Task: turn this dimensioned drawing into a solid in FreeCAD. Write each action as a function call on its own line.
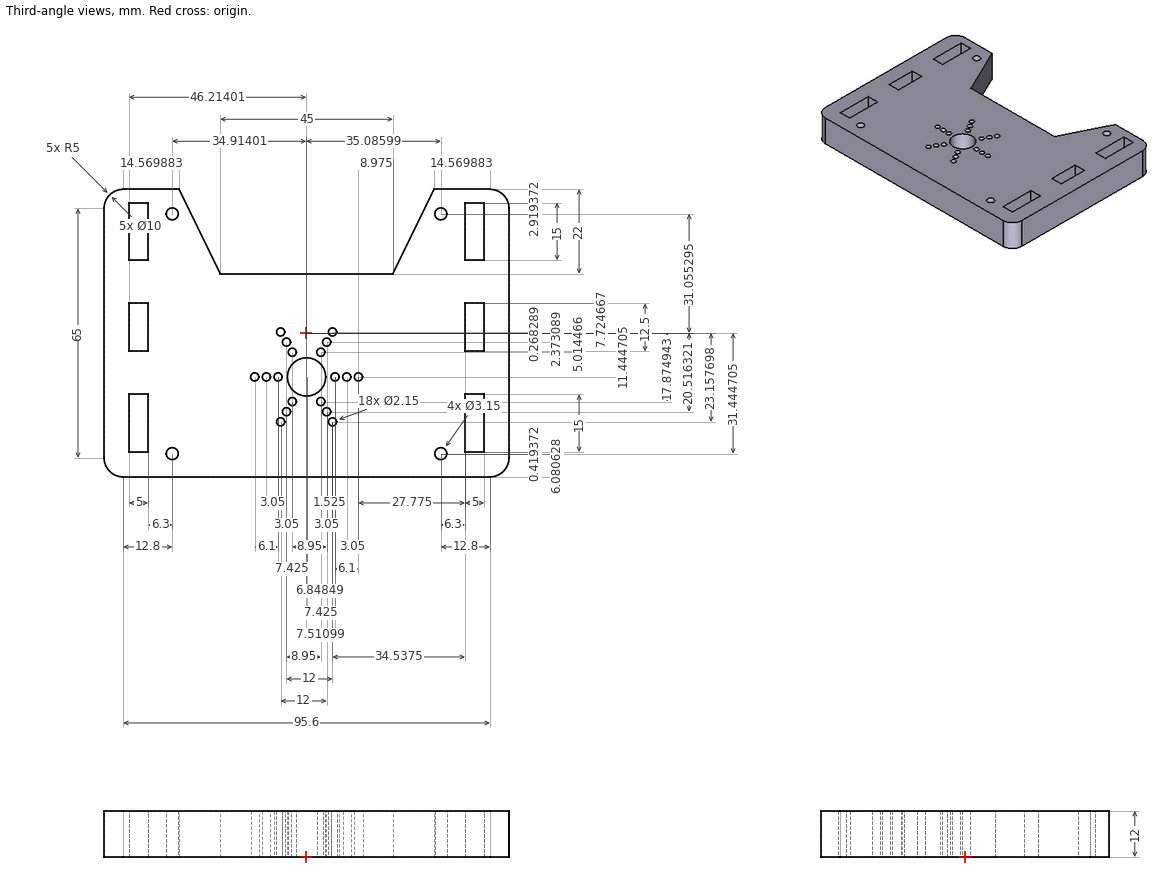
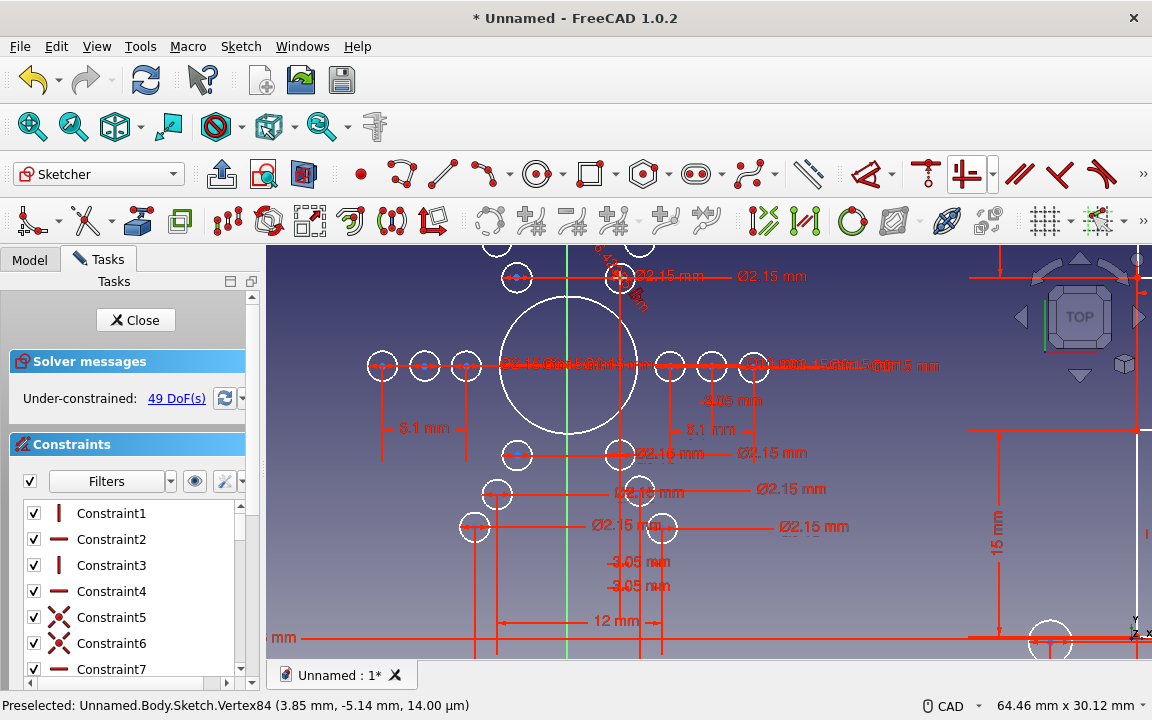
scroll(664, 532, down, 7)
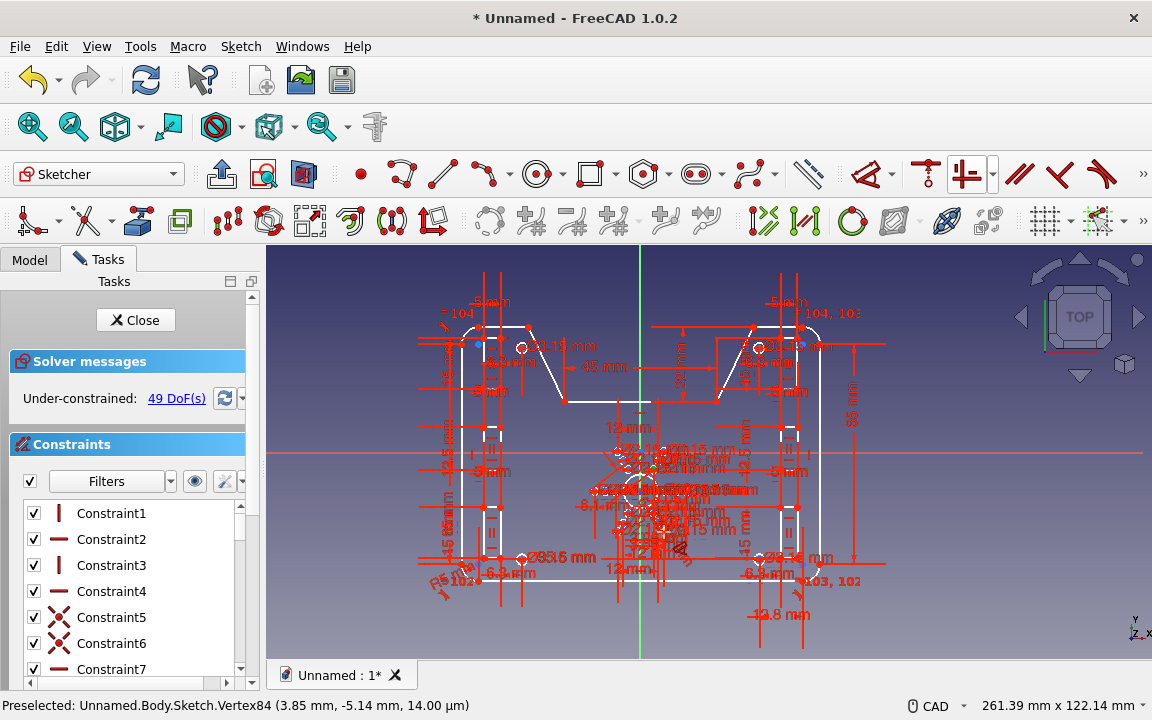
scroll(664, 452, up, 7)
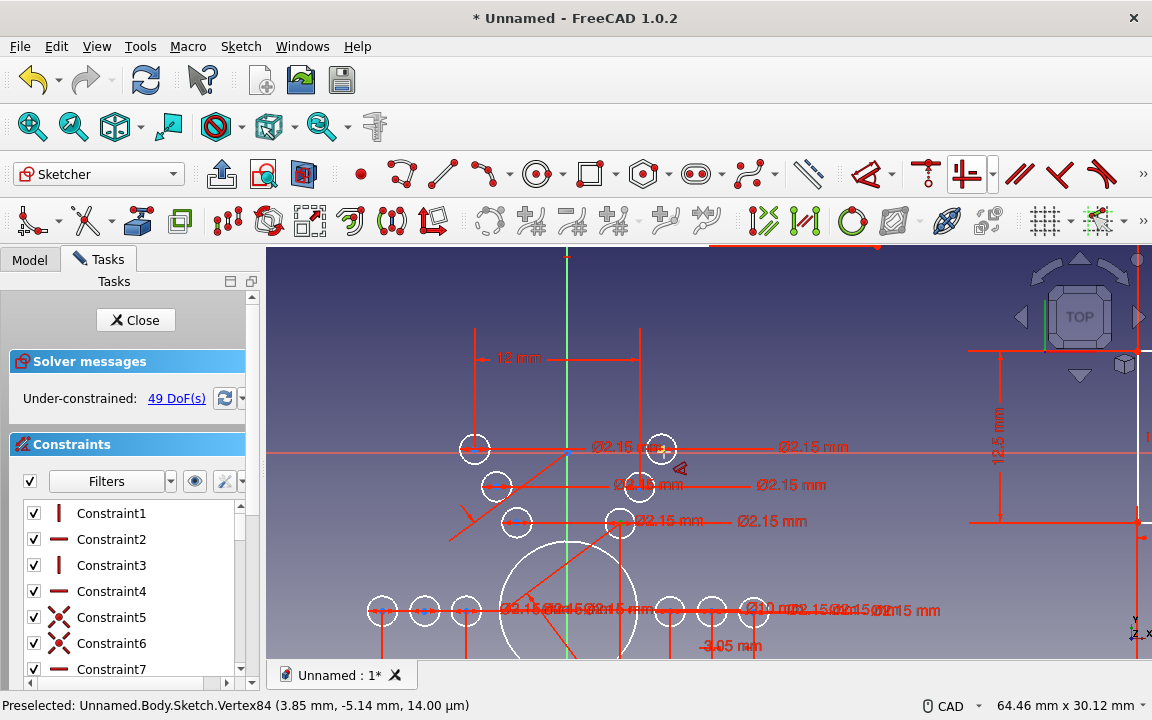
click(661, 449)
click(641, 557)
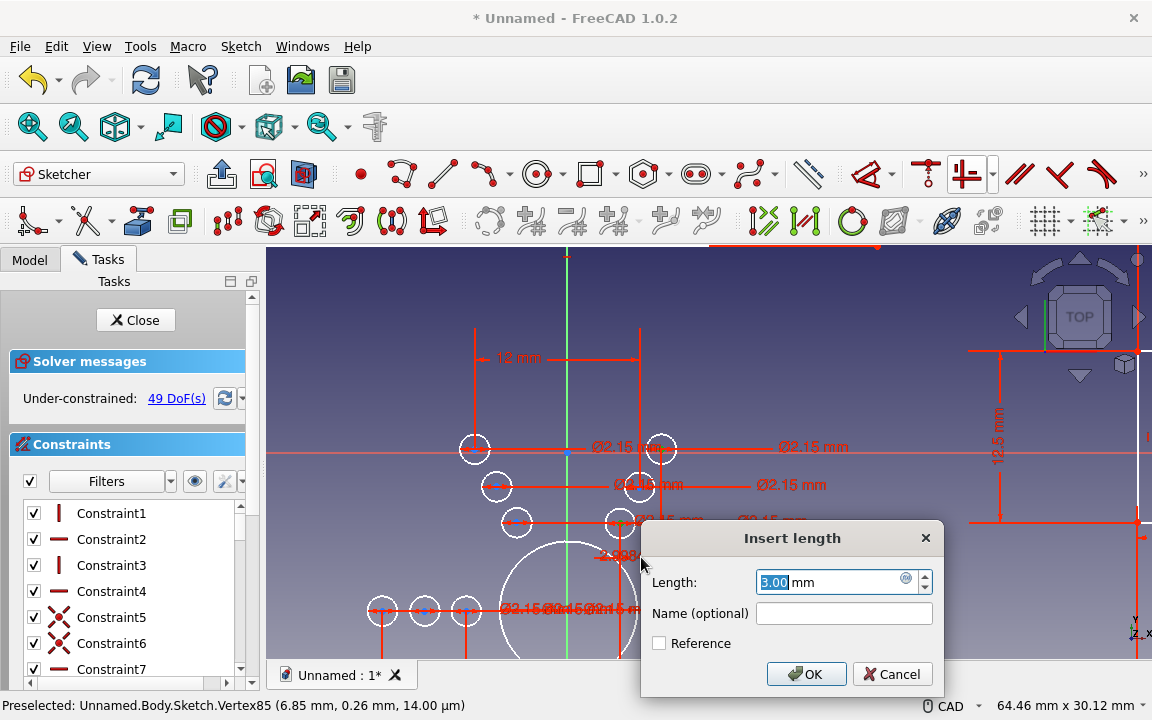
text(3.05)
key(Return)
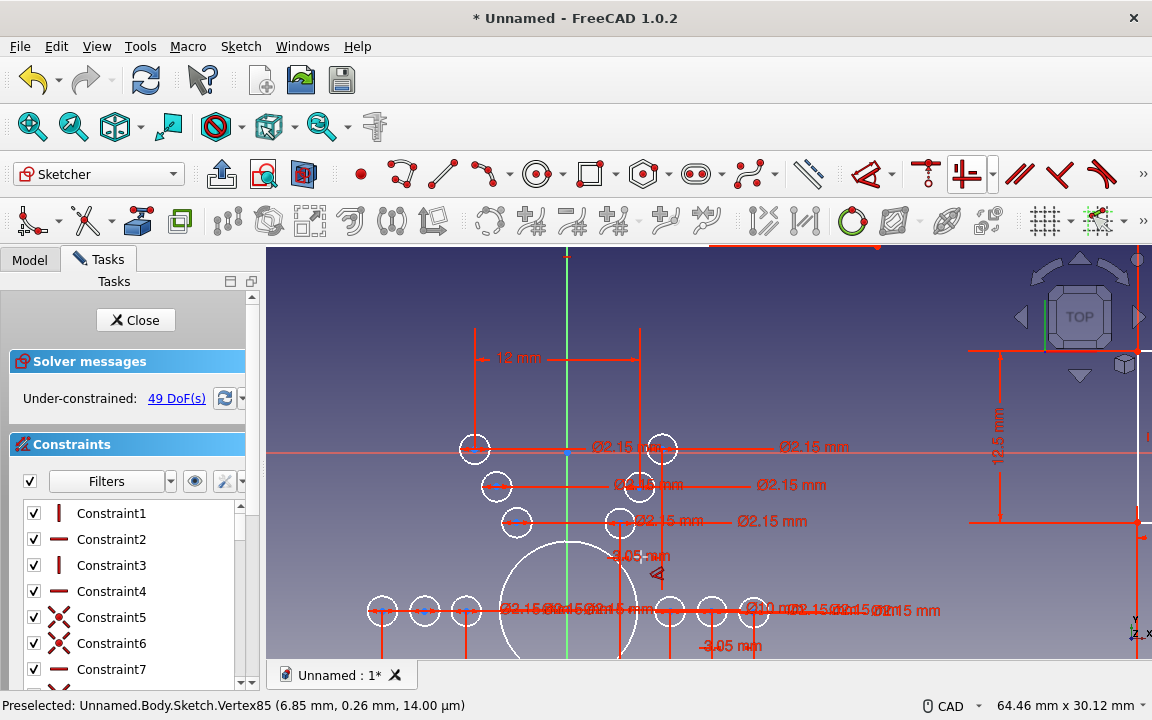
scroll(664, 452, down, 7)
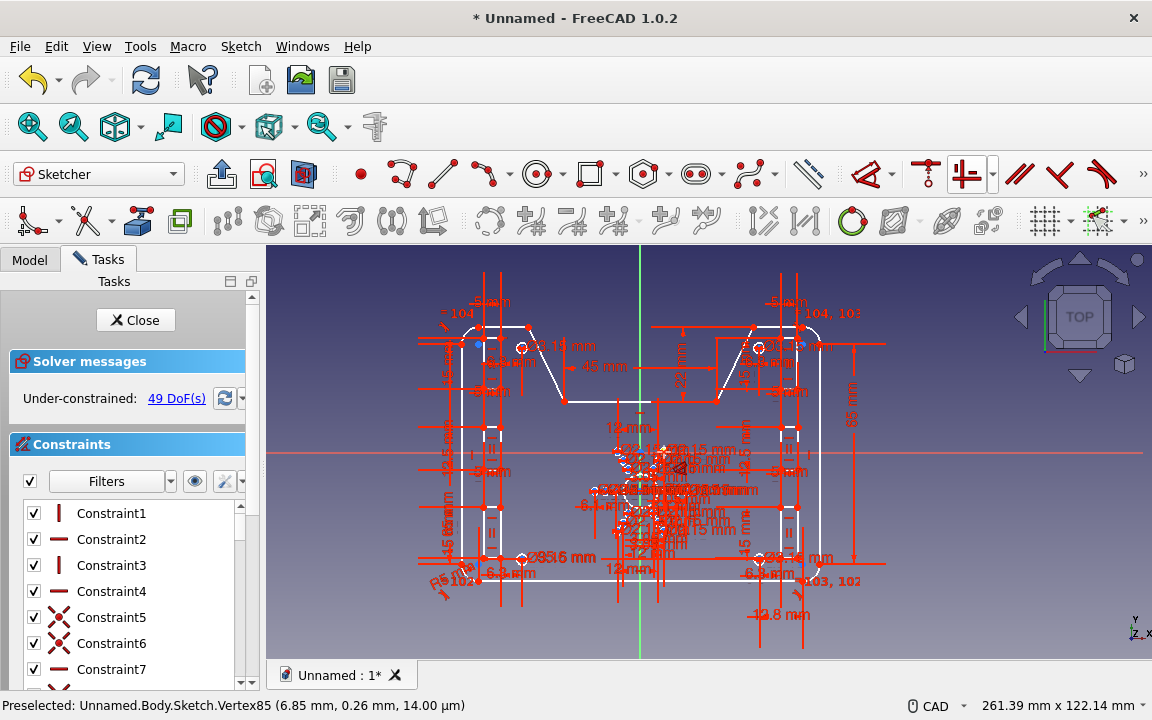
scroll(618, 531, up, 7)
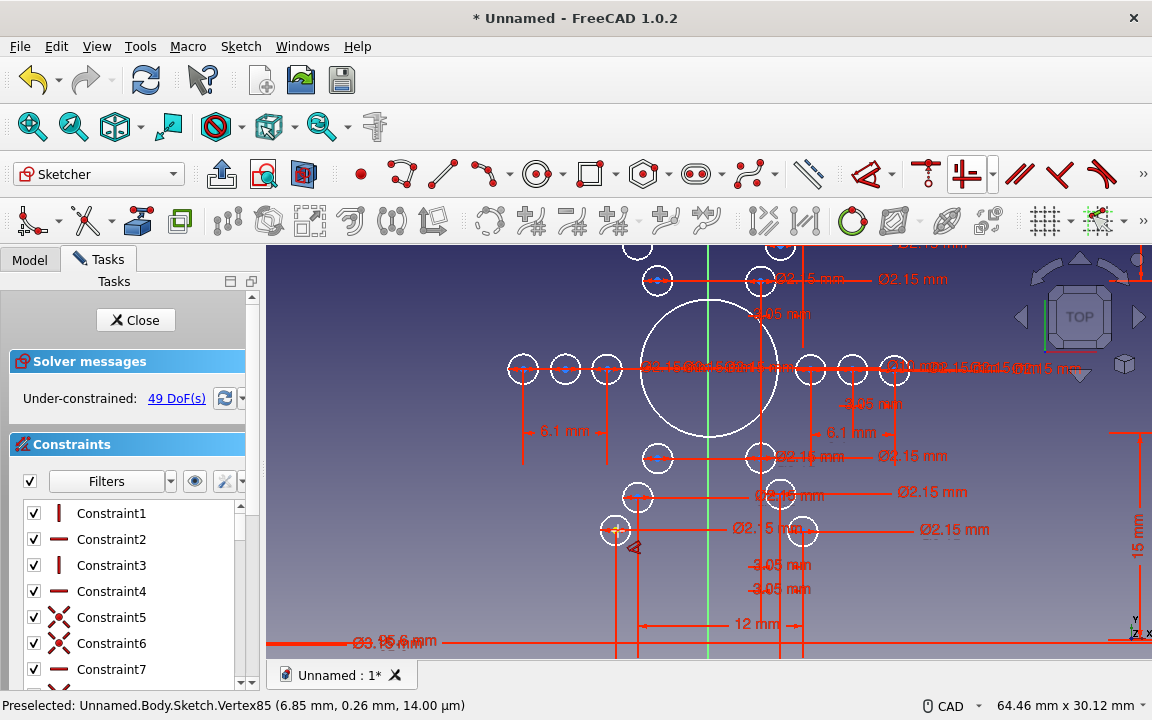
click(616, 530)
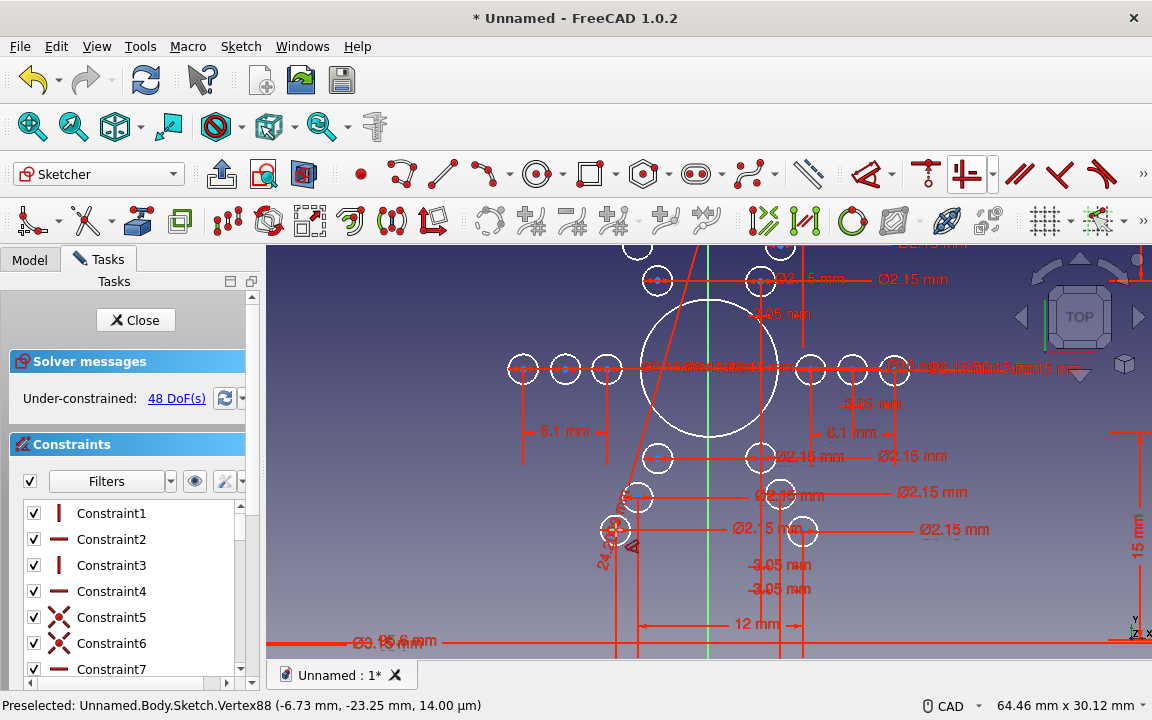
click(658, 459)
click(637, 564)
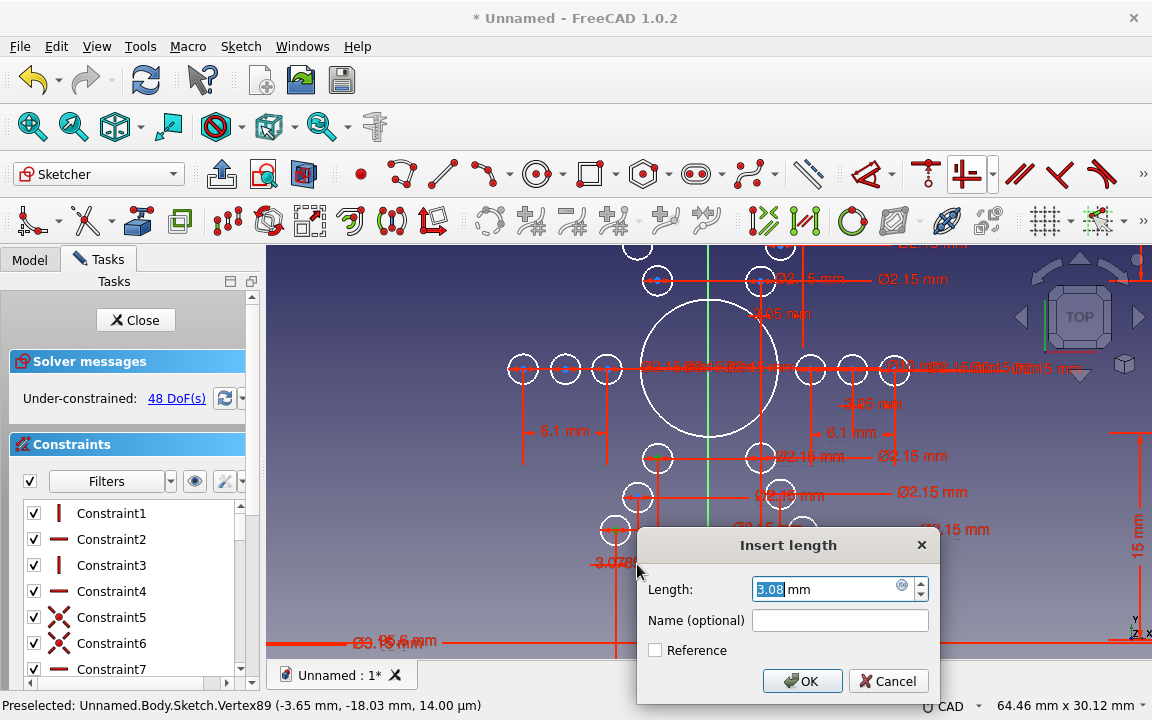
text(3.05)
key(Return)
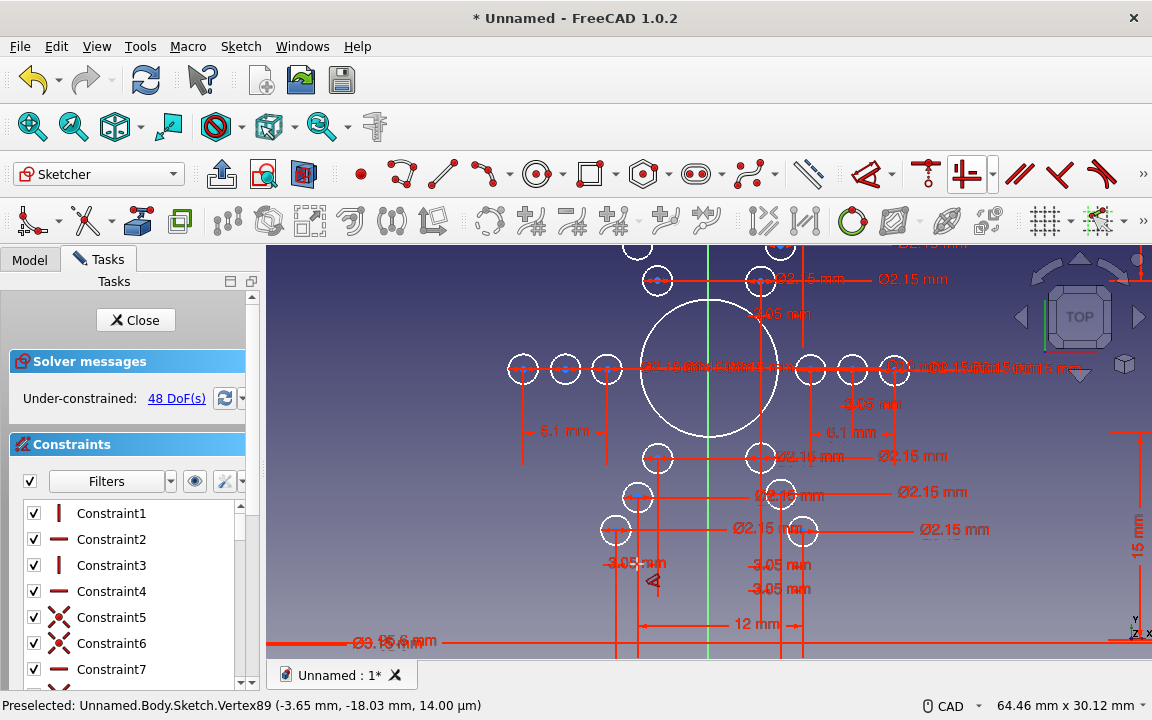
scroll(618, 531, down, 7)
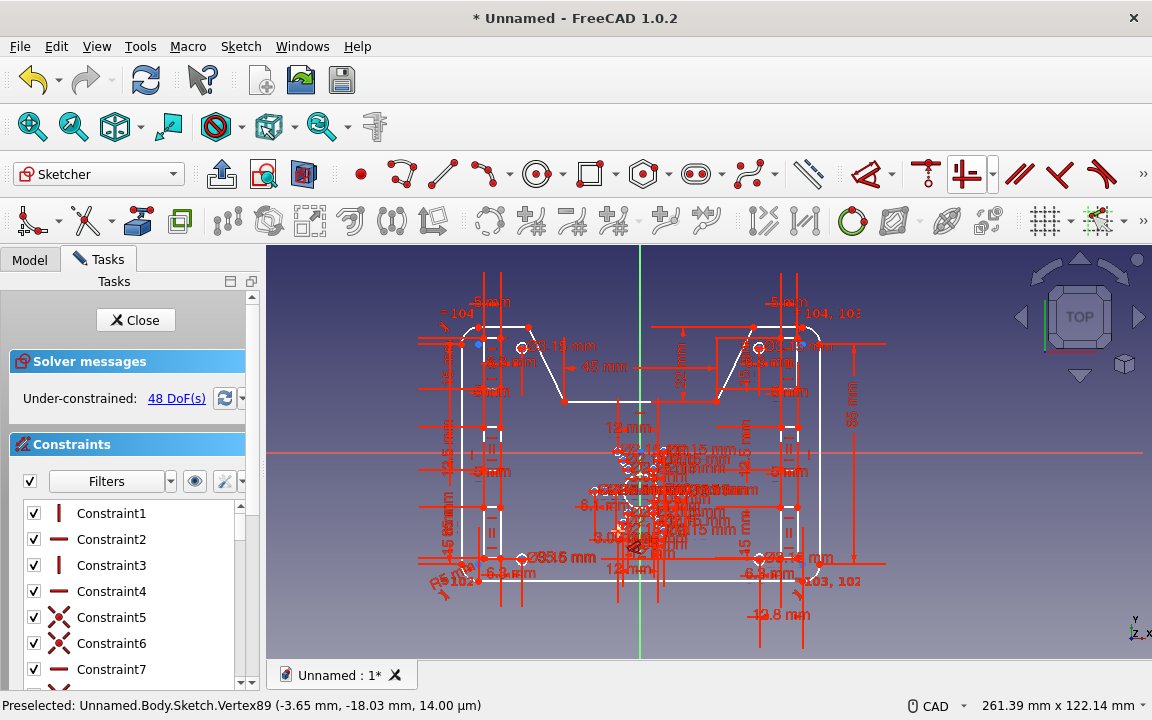
click(479, 581)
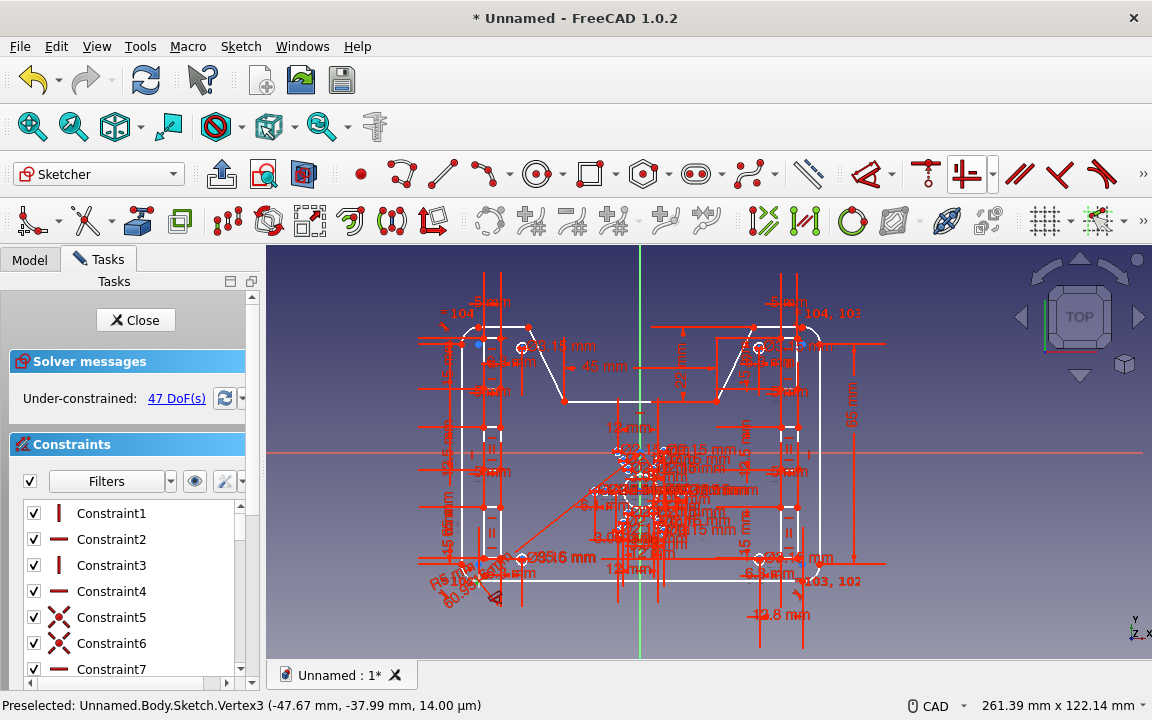
click(522, 560)
click(501, 615)